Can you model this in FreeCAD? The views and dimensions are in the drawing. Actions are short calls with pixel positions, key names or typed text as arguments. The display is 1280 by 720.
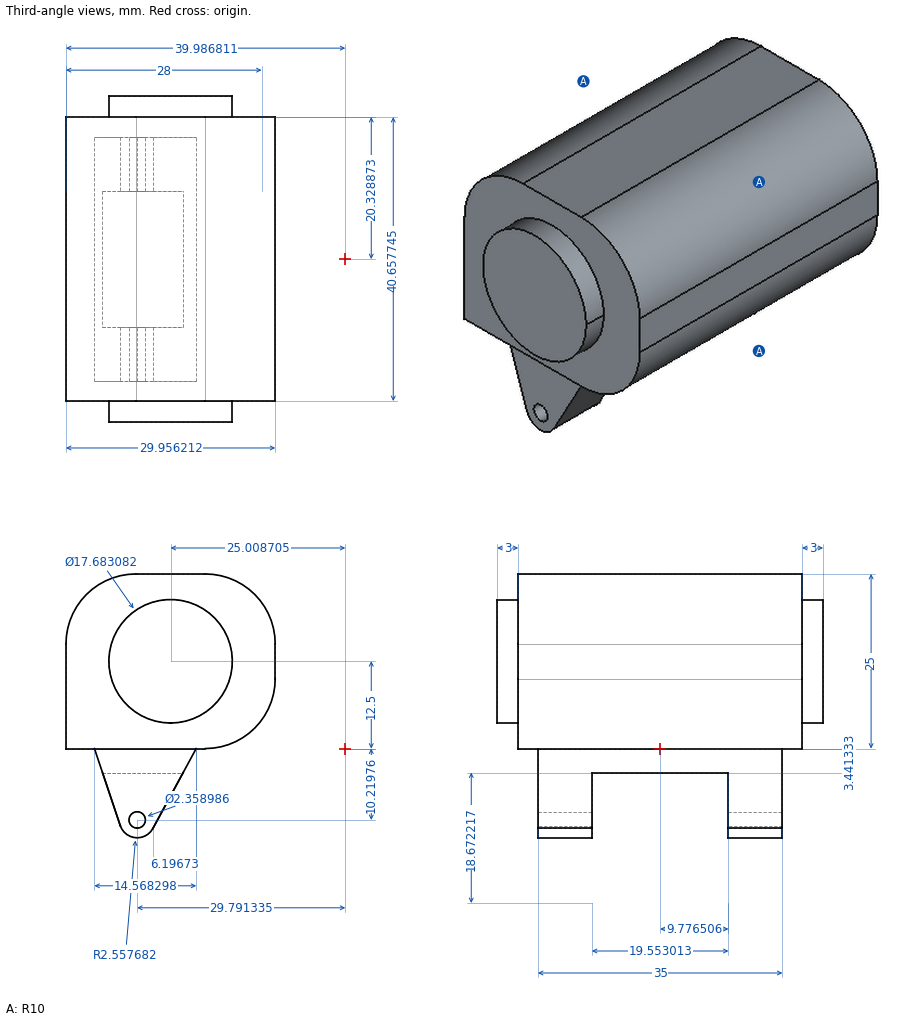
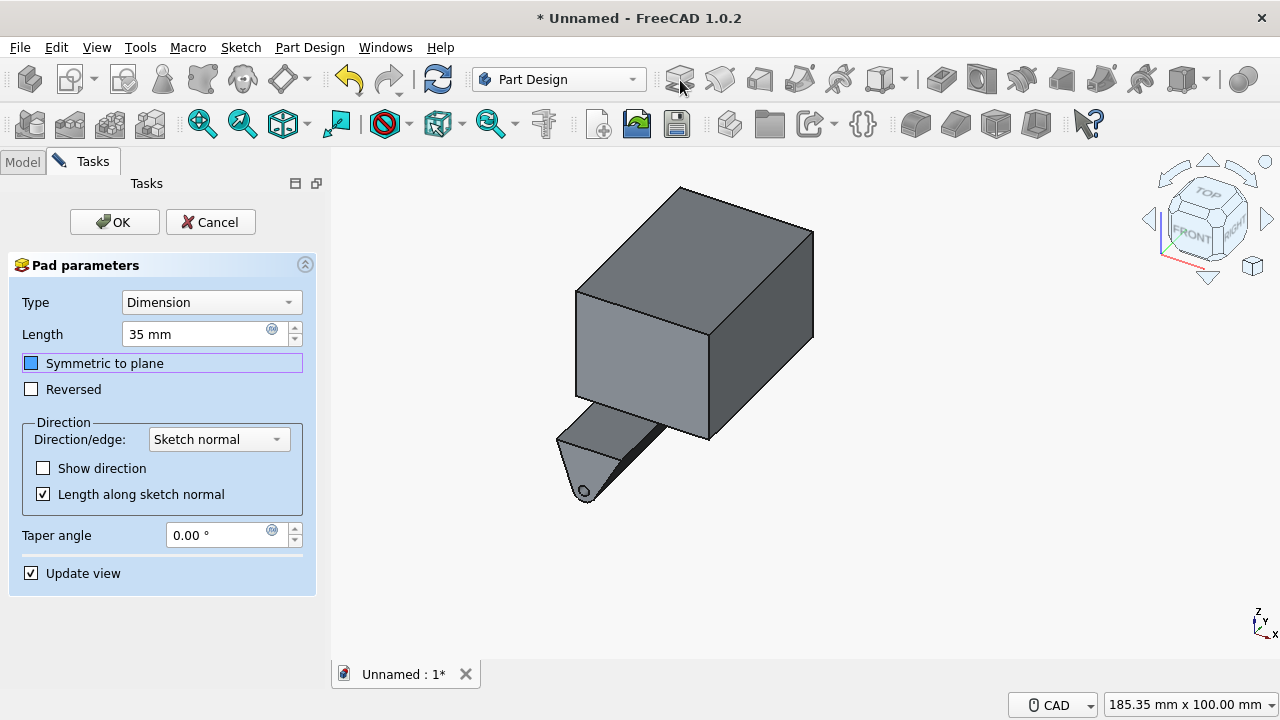
click(30, 363)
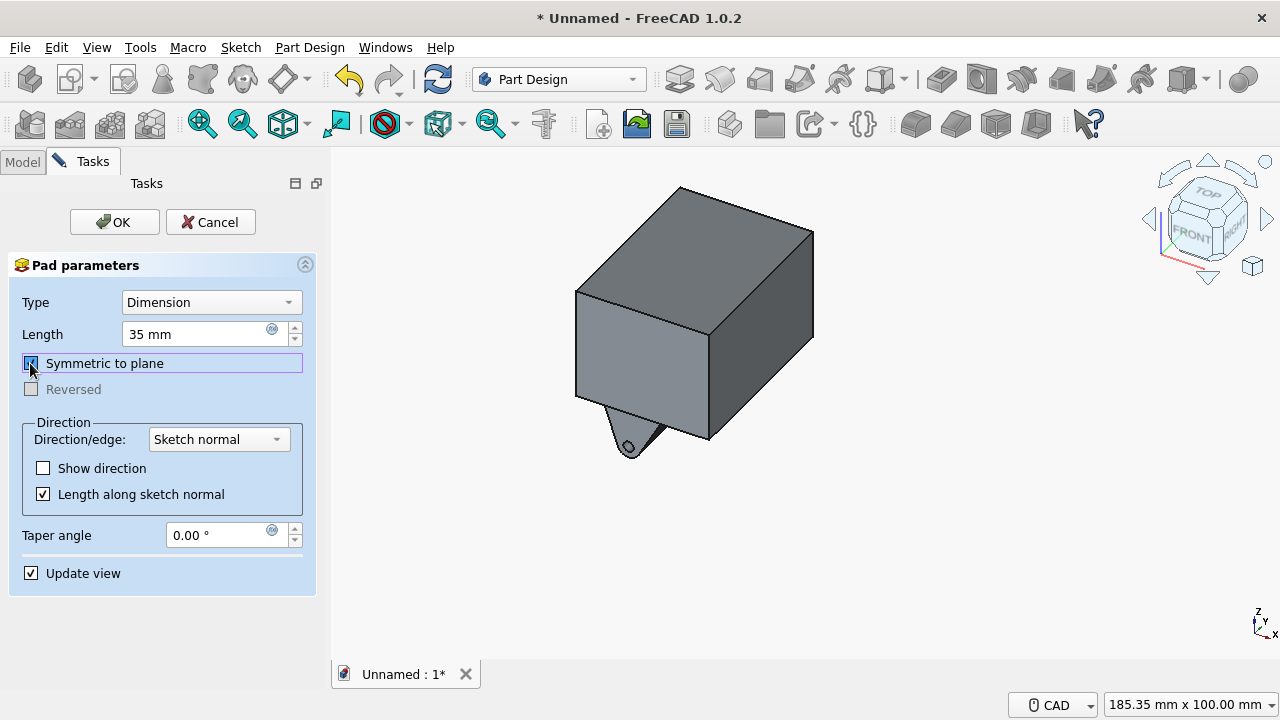
click(115, 222)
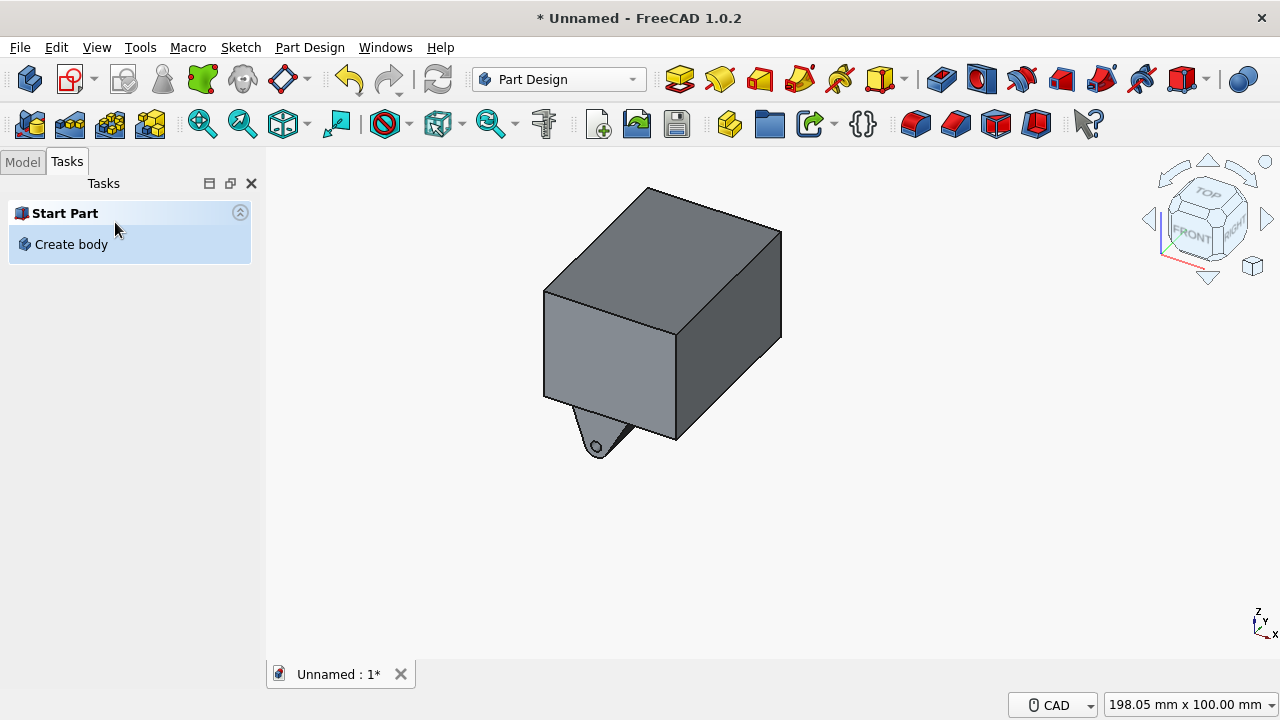
click(729, 282)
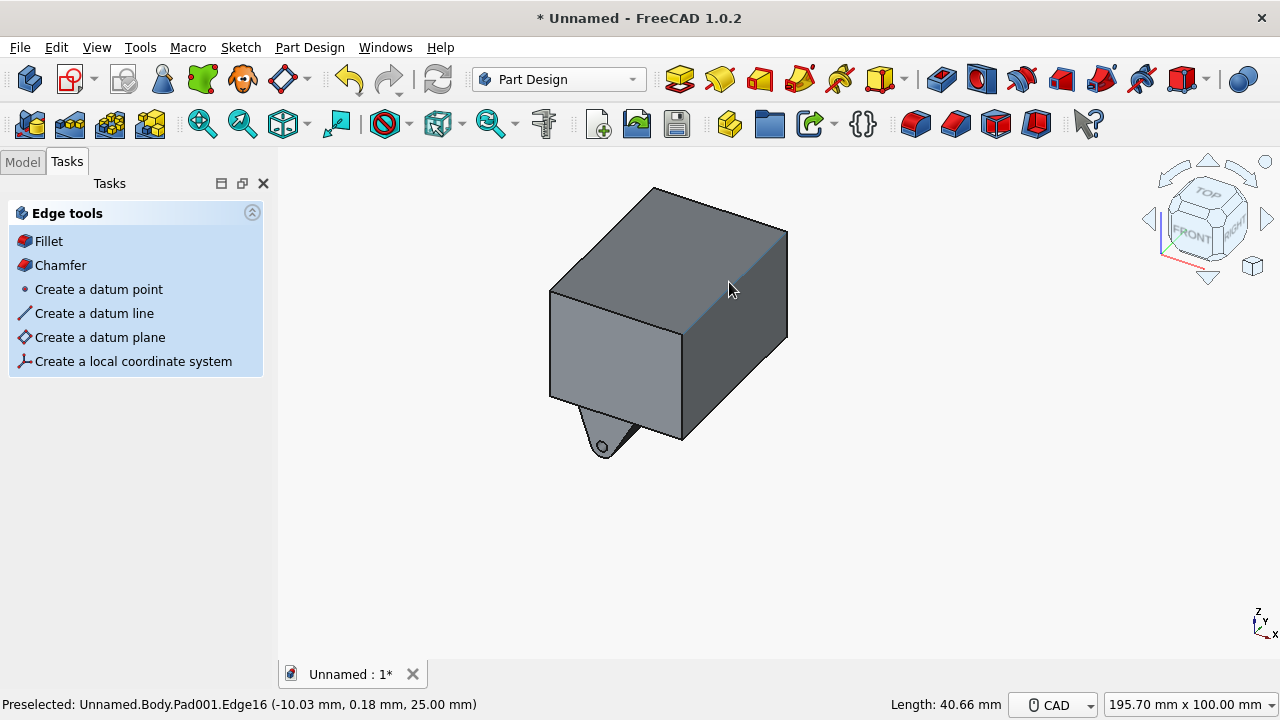
key(0)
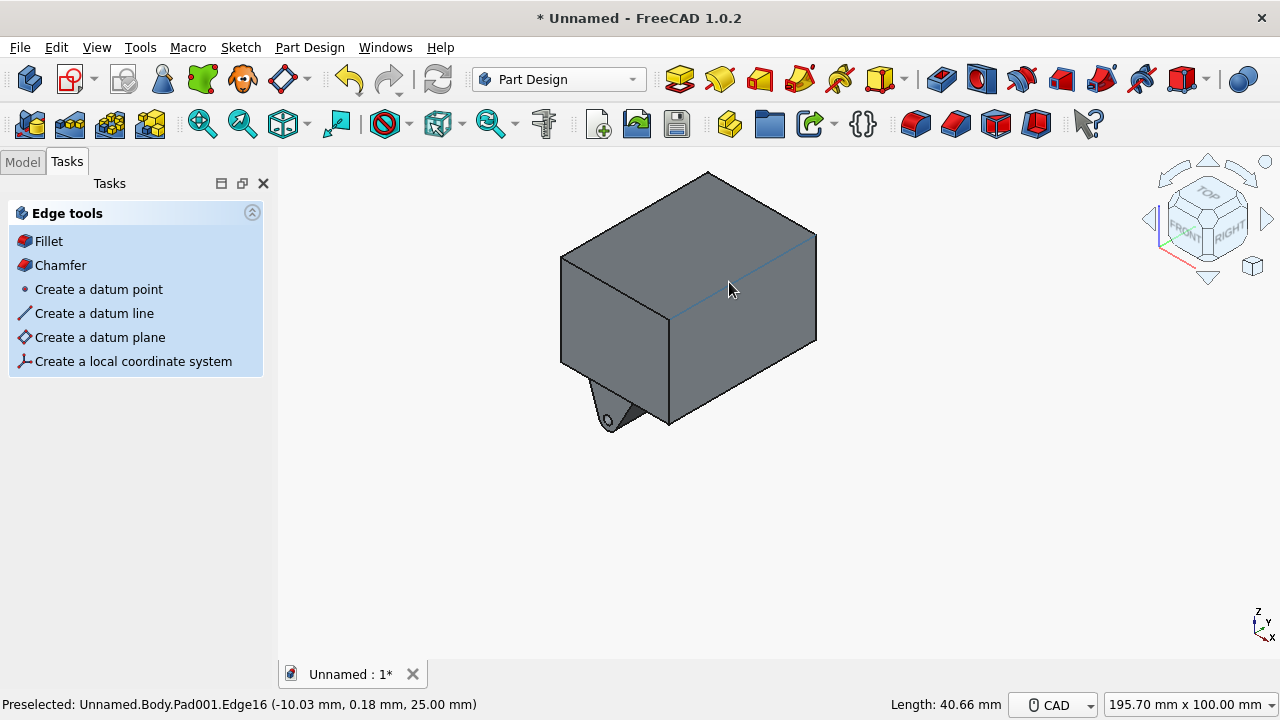
key(2)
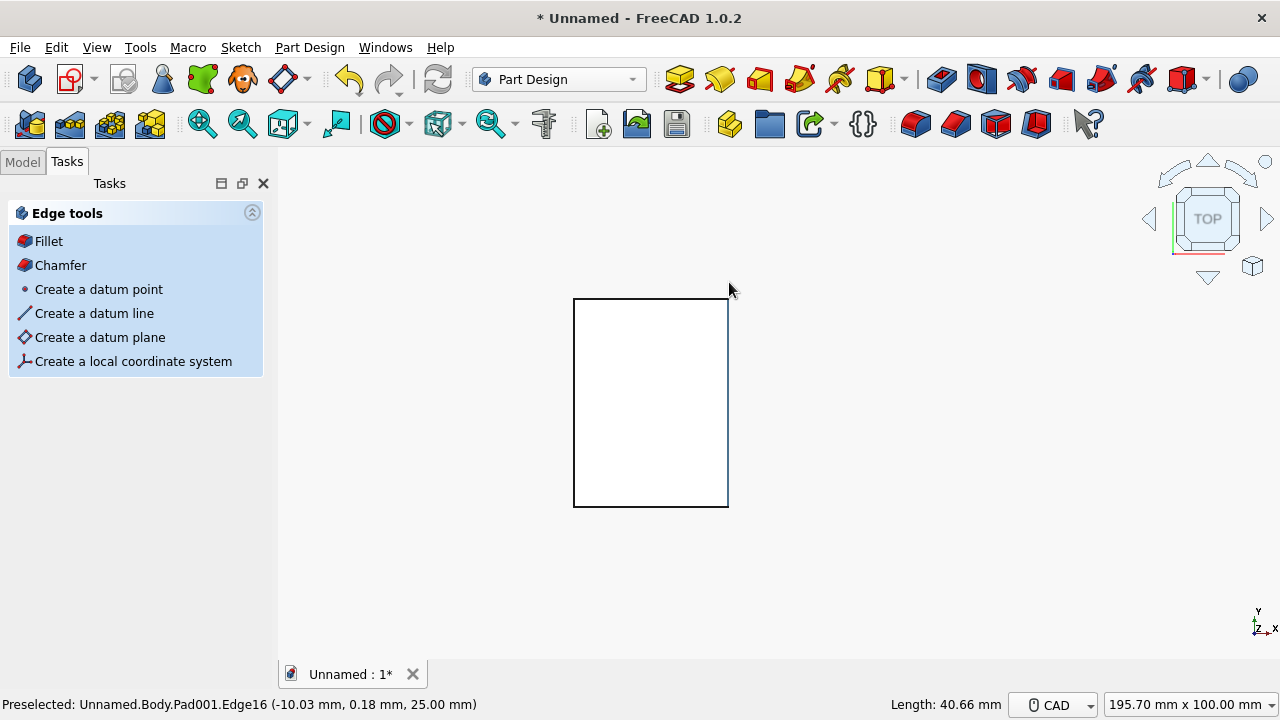
click(204, 124)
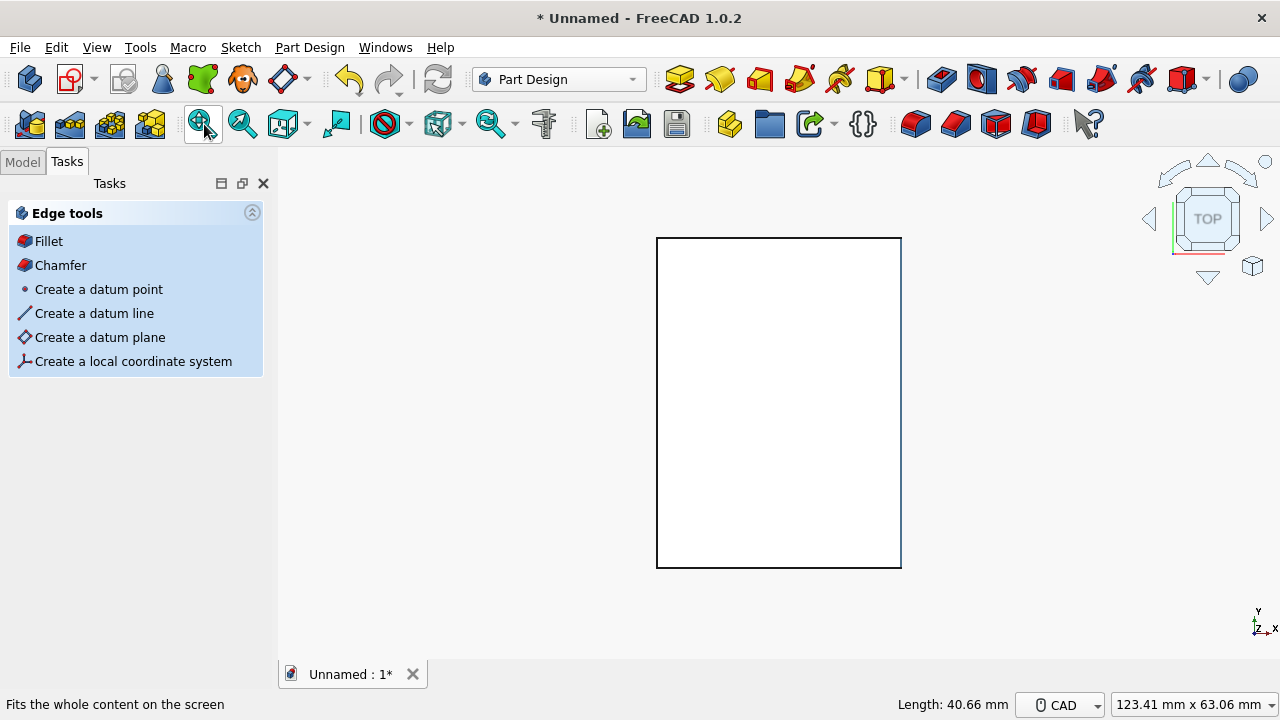
click(657, 402, ctrl)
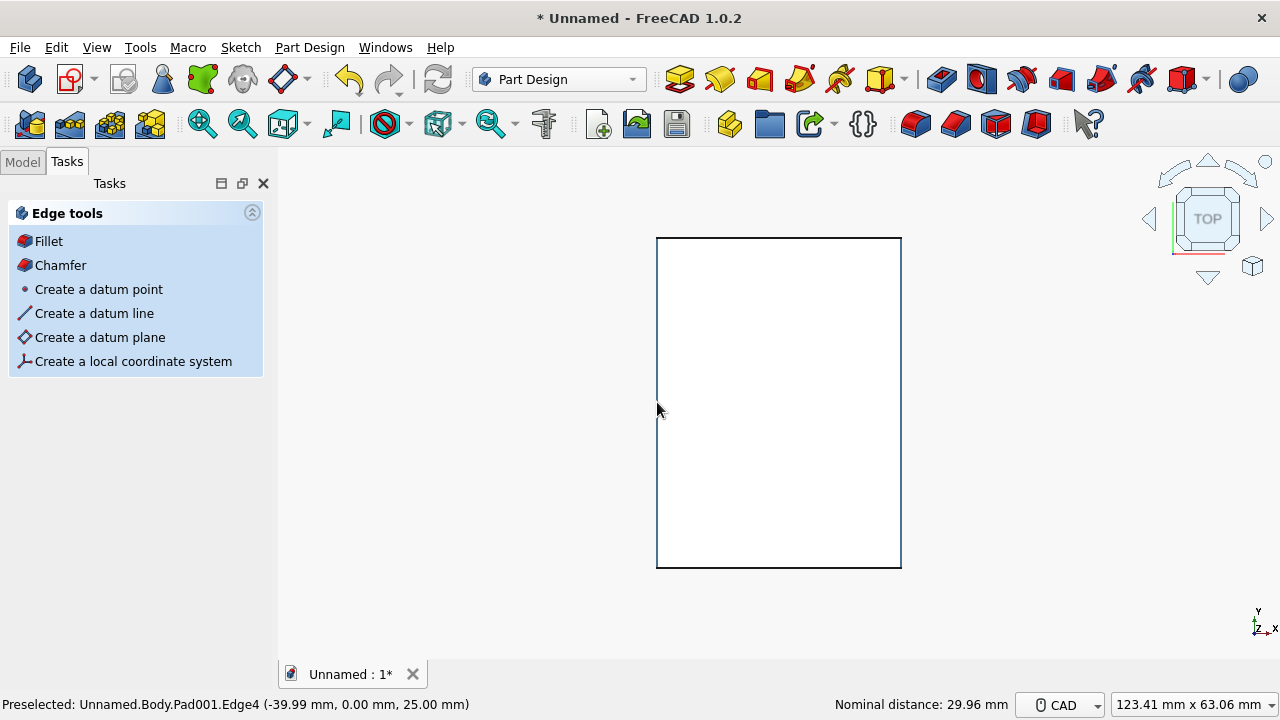
key(1)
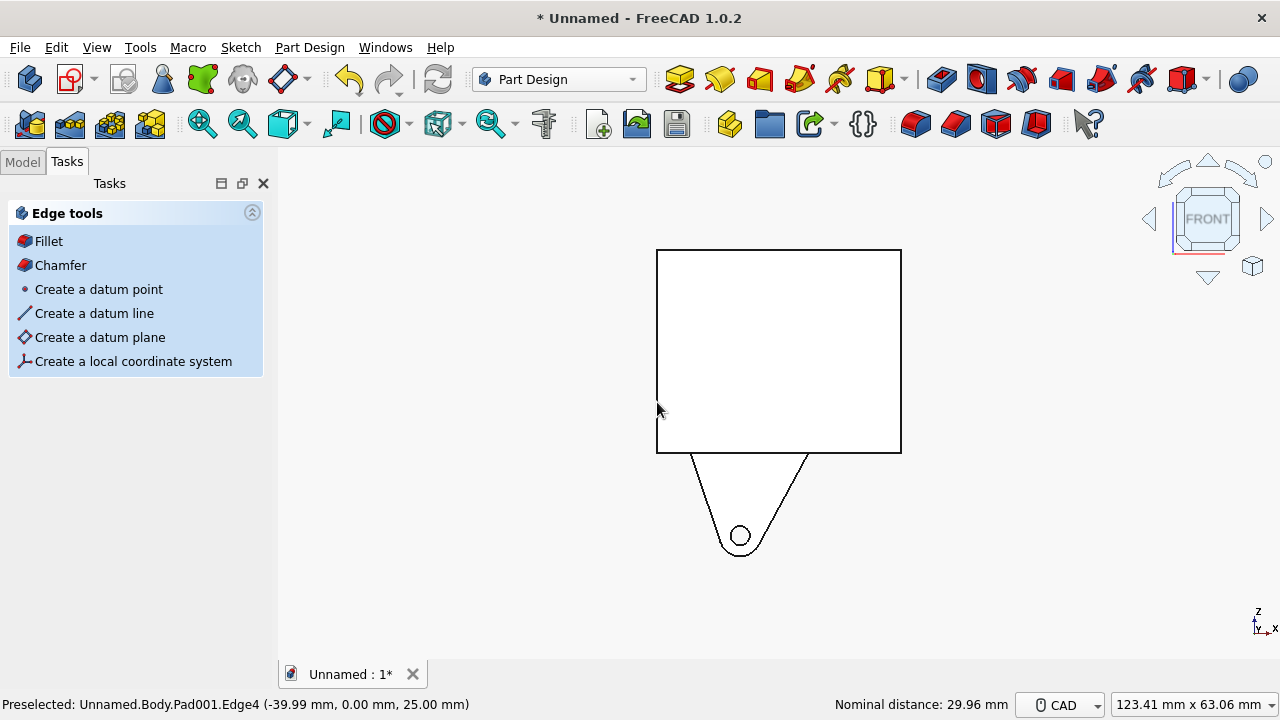
key(3)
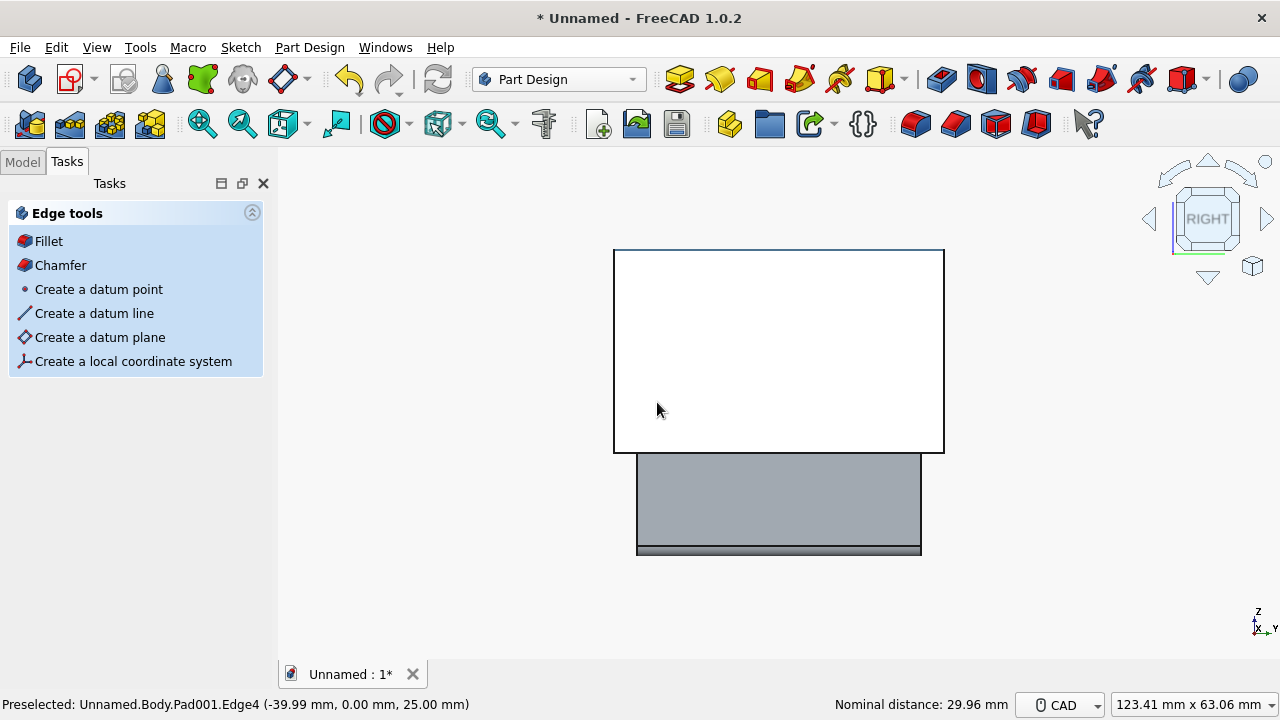
click(779, 452, ctrl)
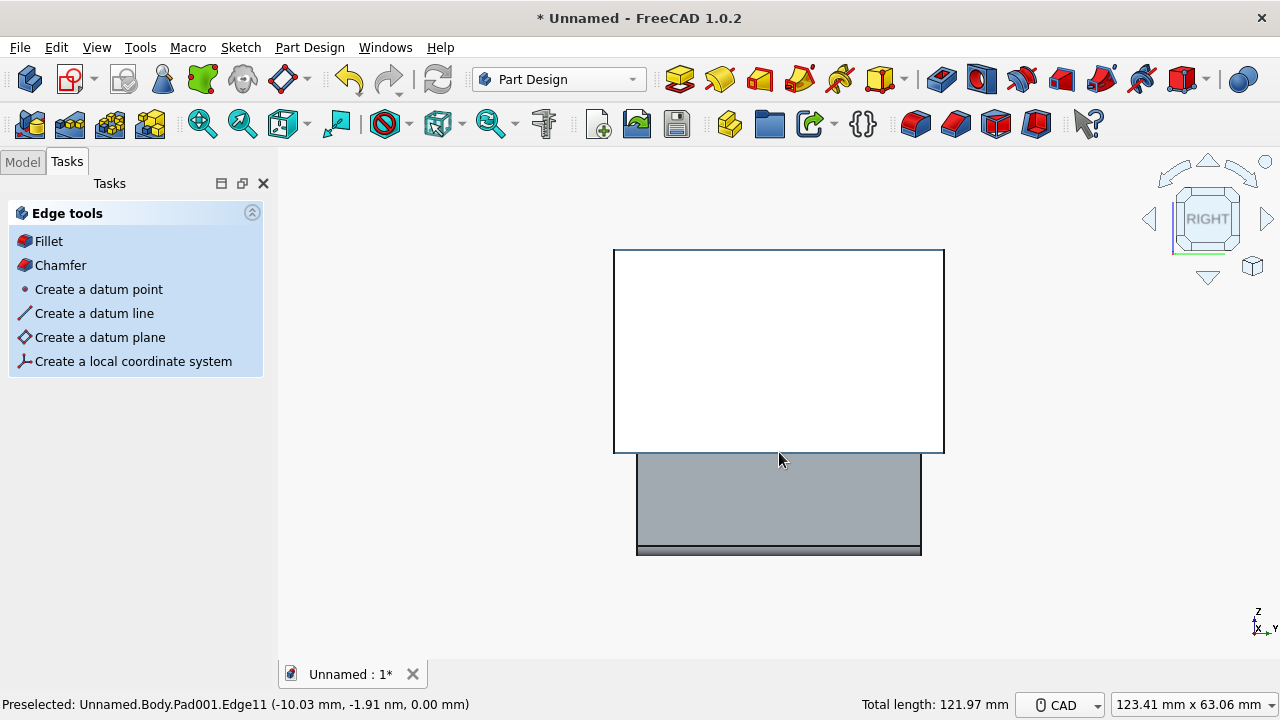
click(916, 124)